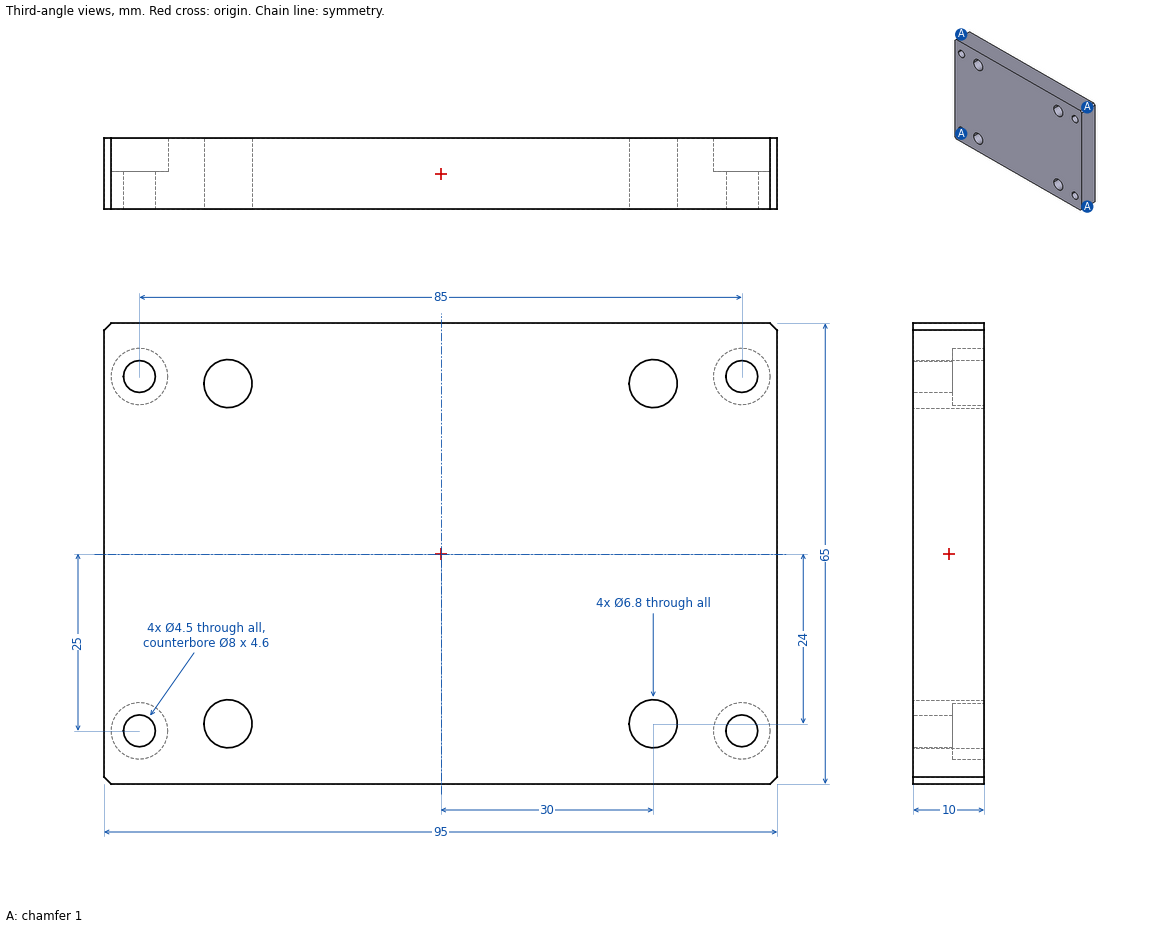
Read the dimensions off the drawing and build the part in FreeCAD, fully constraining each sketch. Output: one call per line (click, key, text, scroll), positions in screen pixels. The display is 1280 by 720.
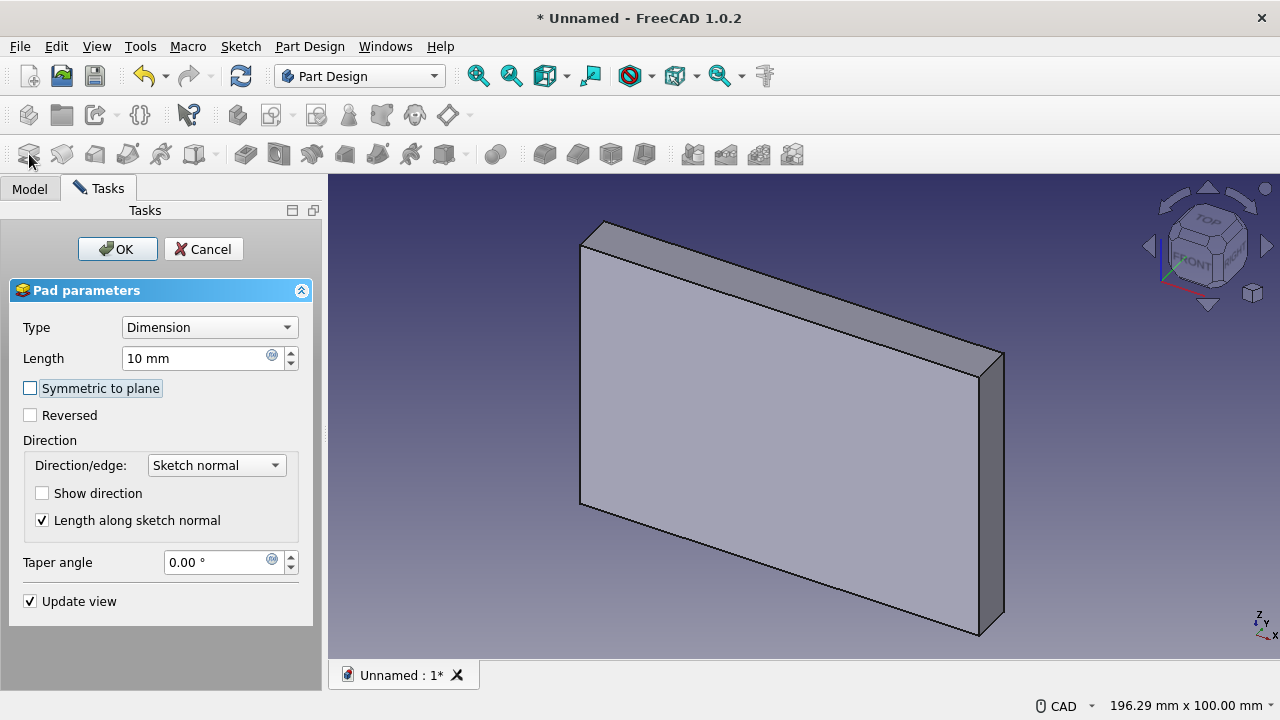
click(31, 388)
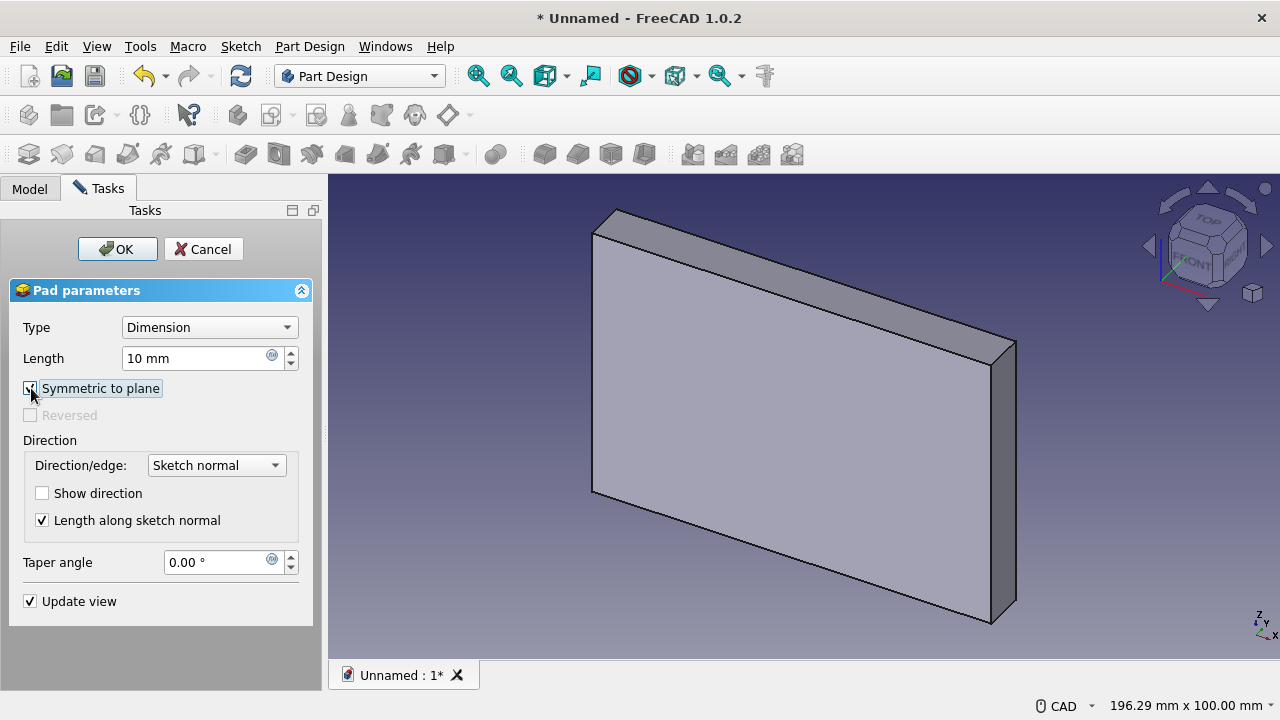
click(118, 249)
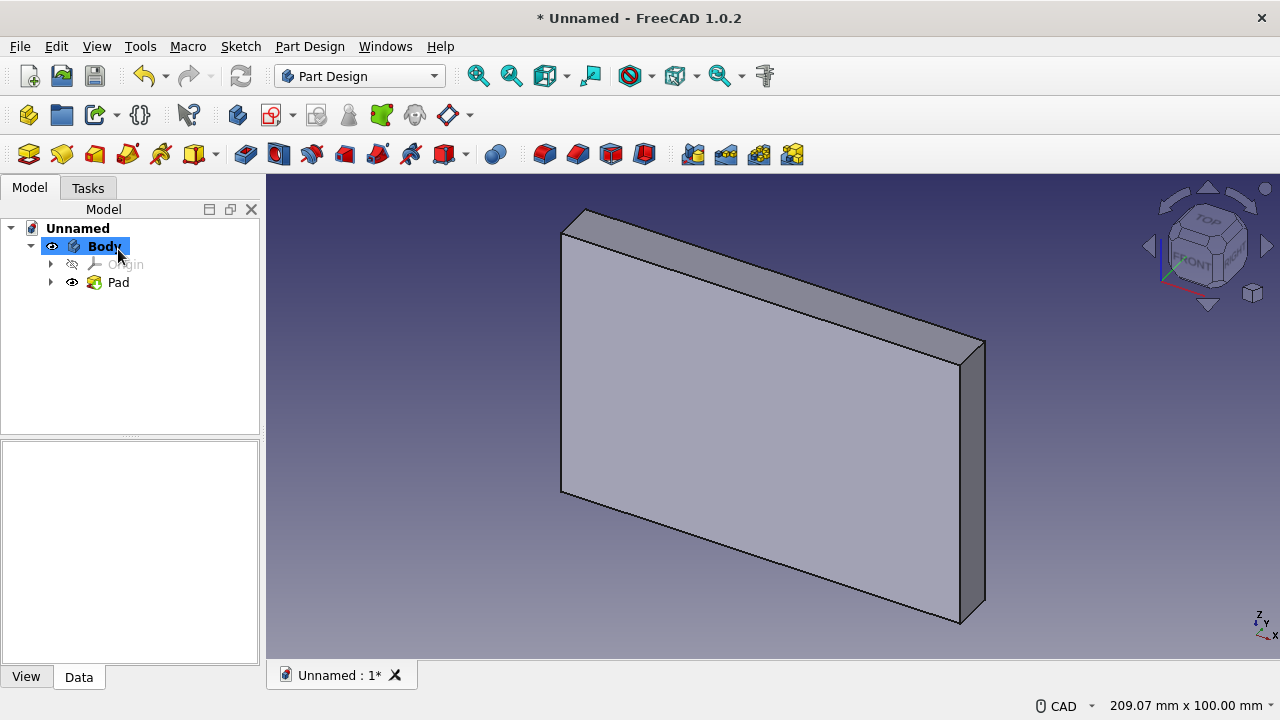
click(973, 352)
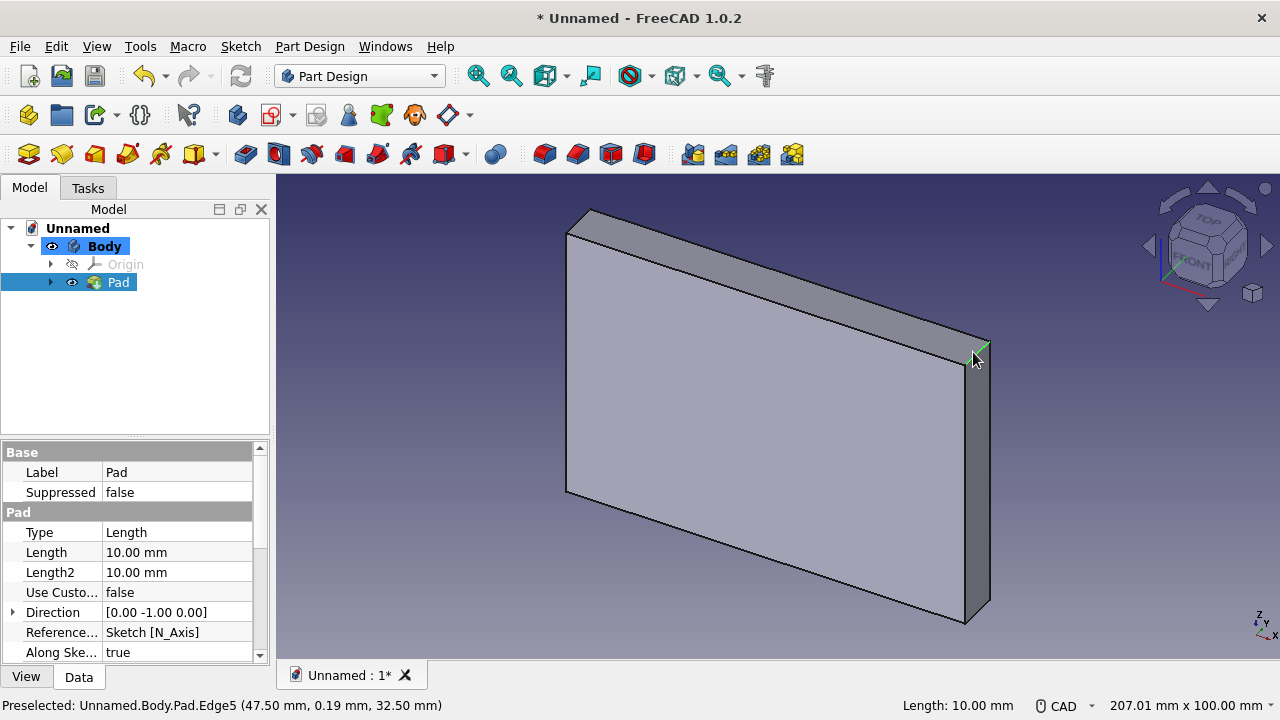
key(0)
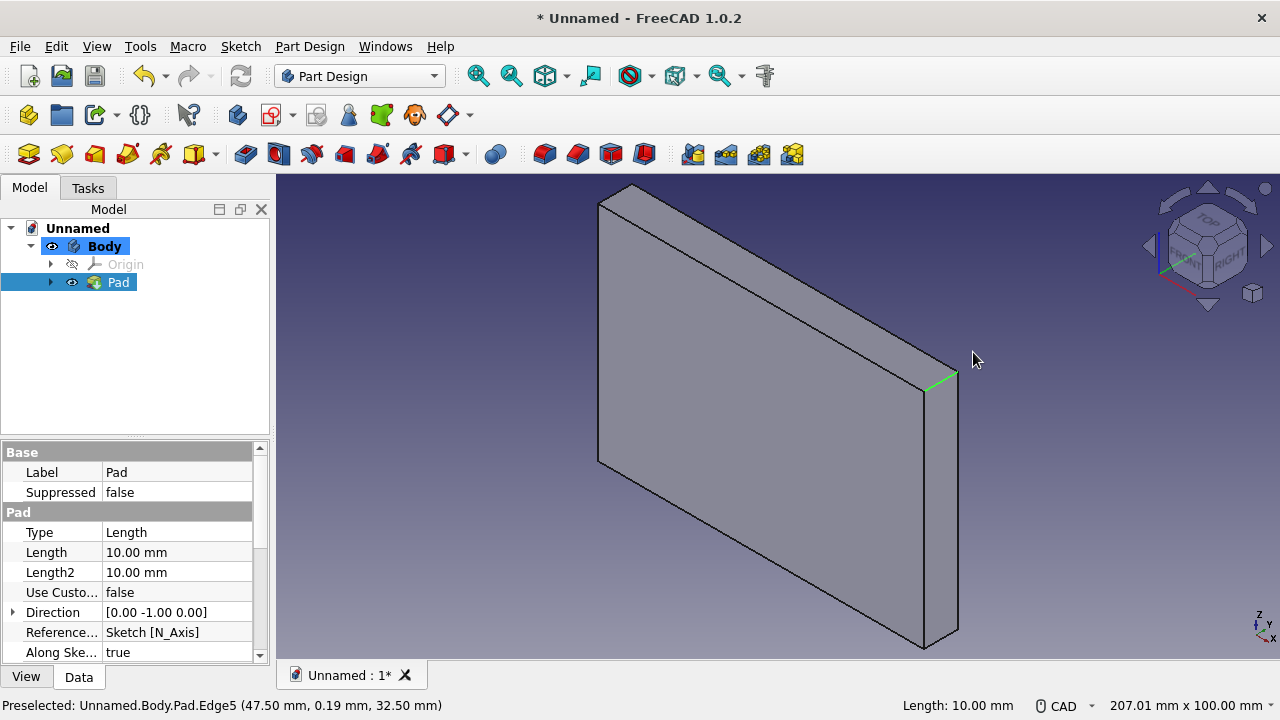
key(2)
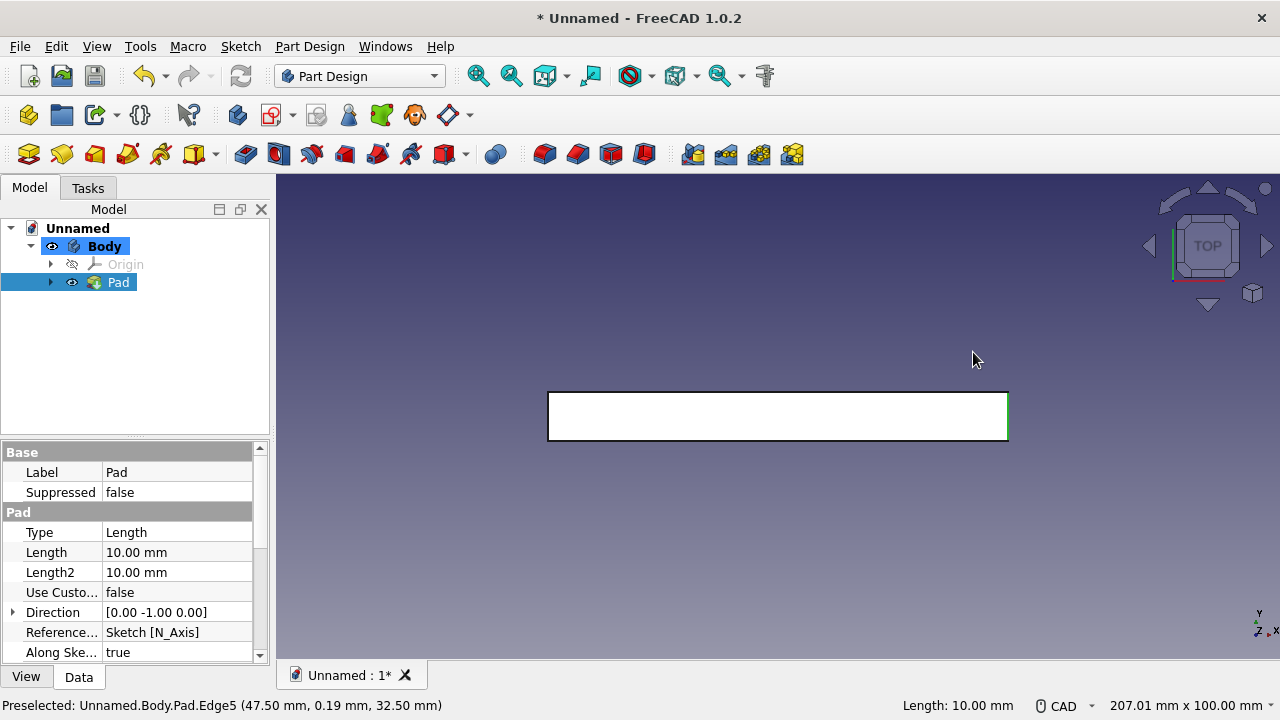
click(548, 415, ctrl)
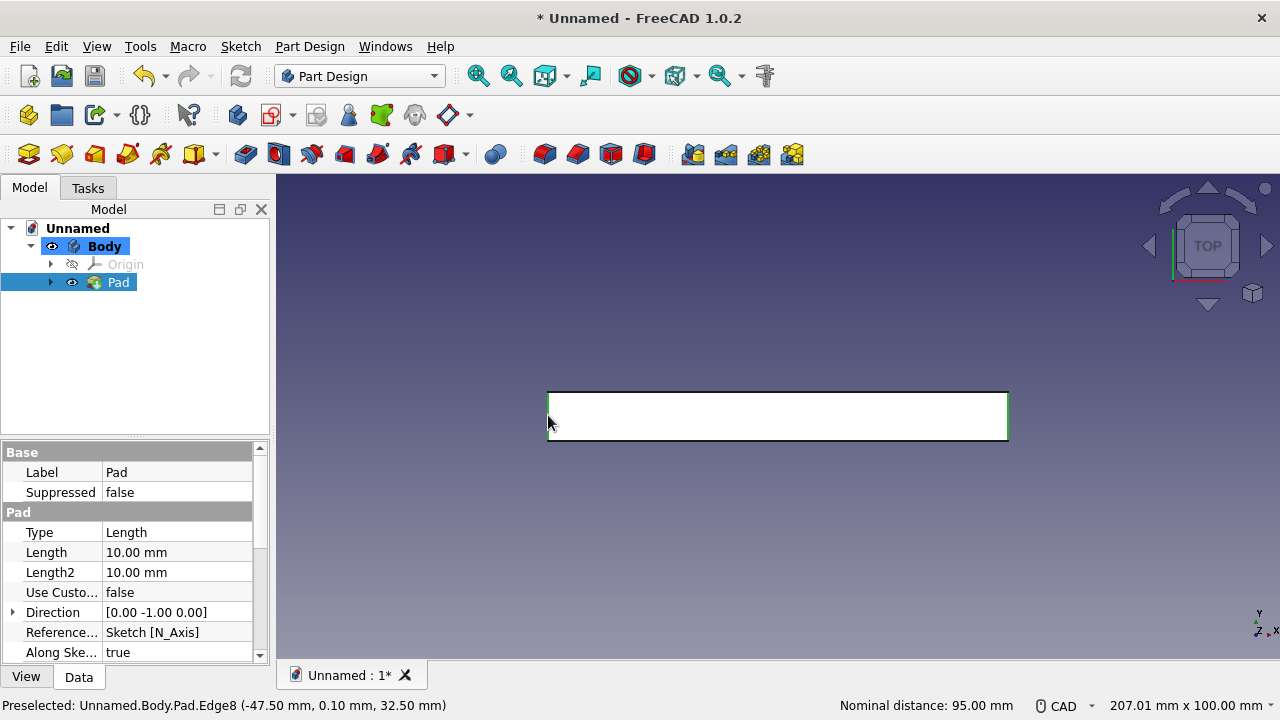
key(1)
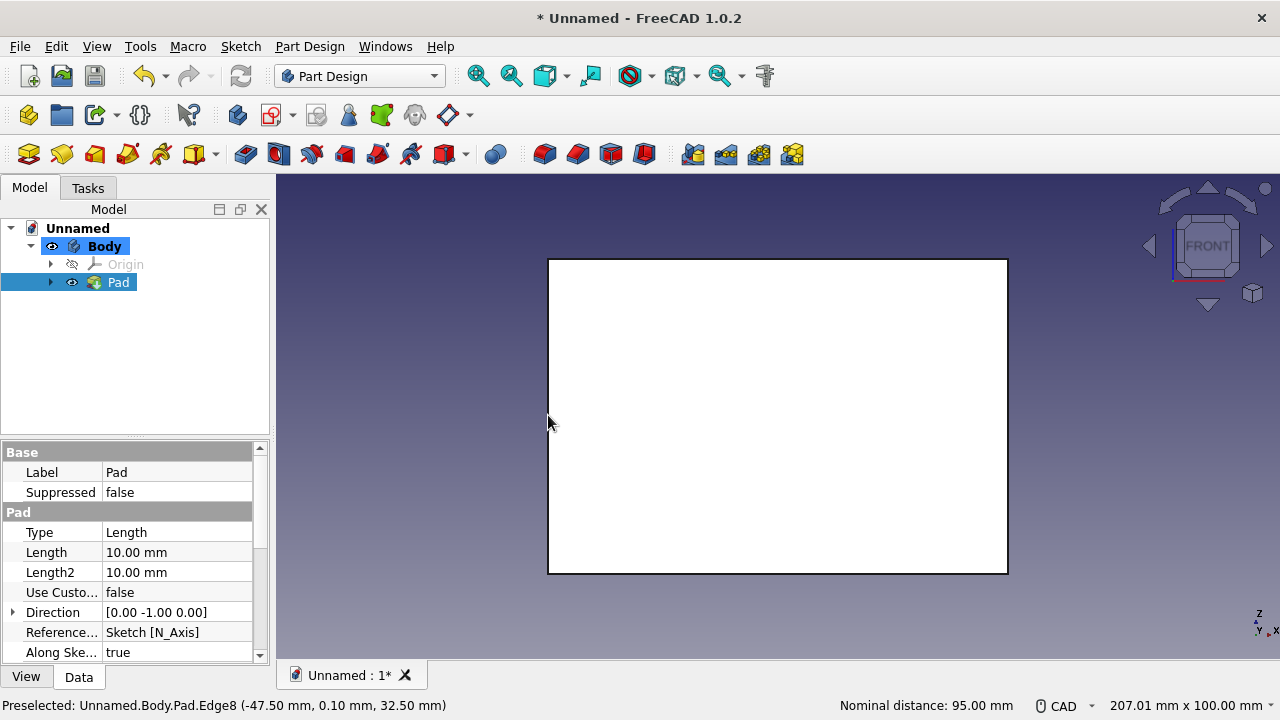
key(3)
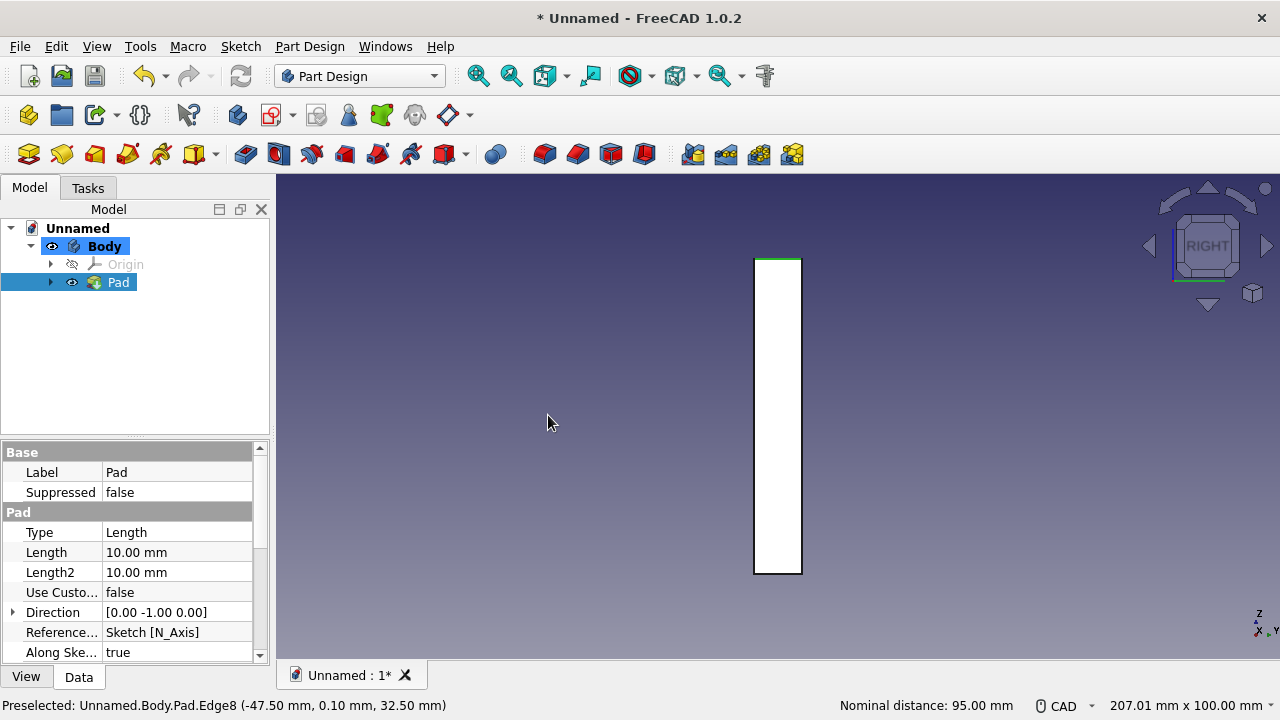
click(778, 573, ctrl)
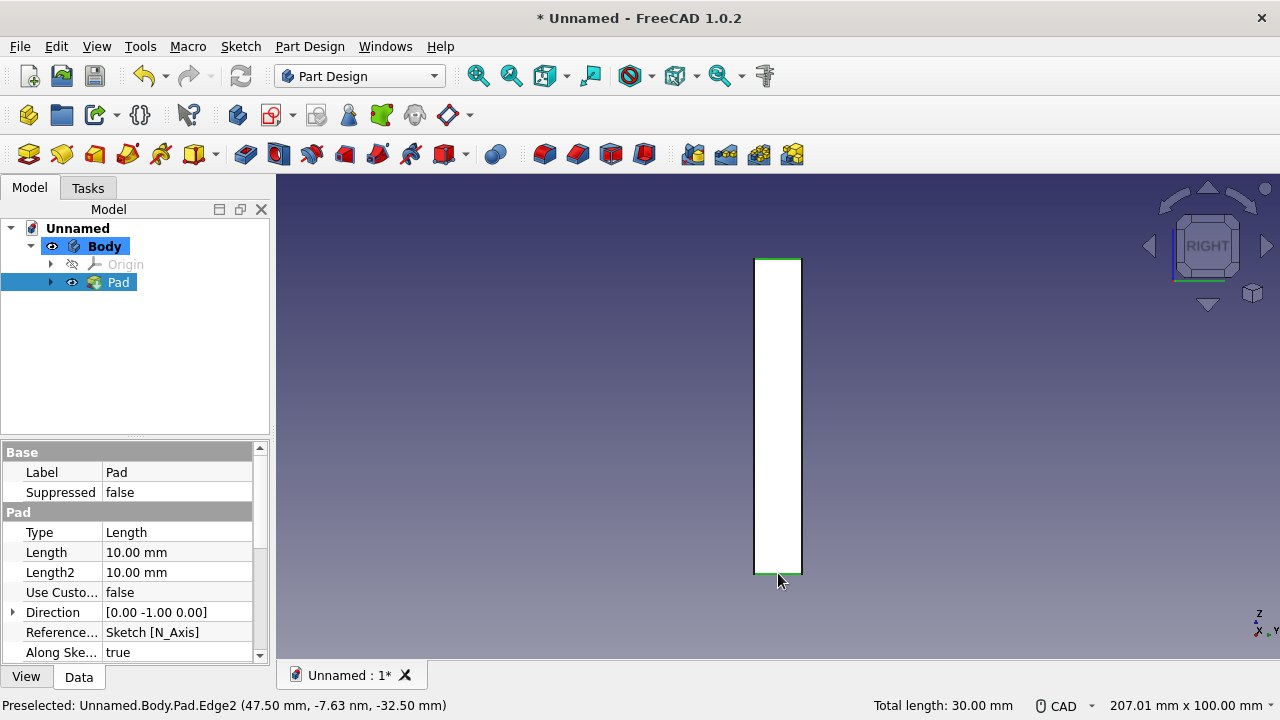
key(5)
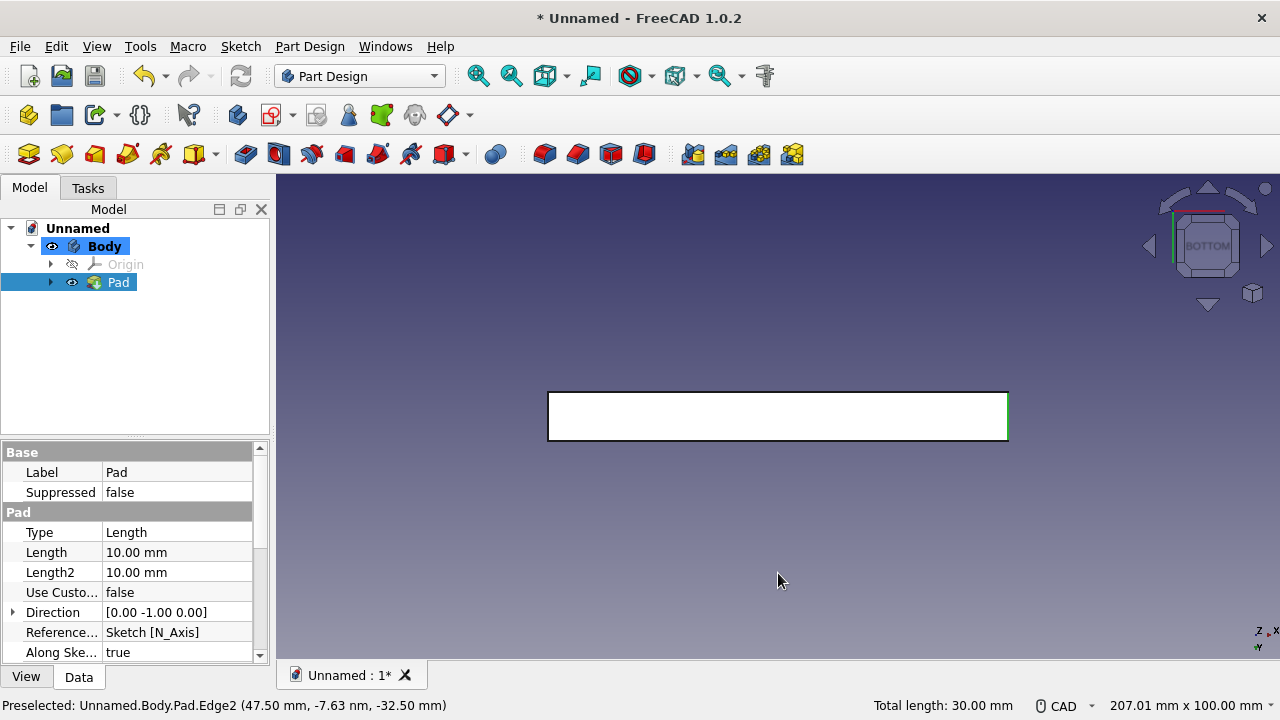
click(548, 416, ctrl)